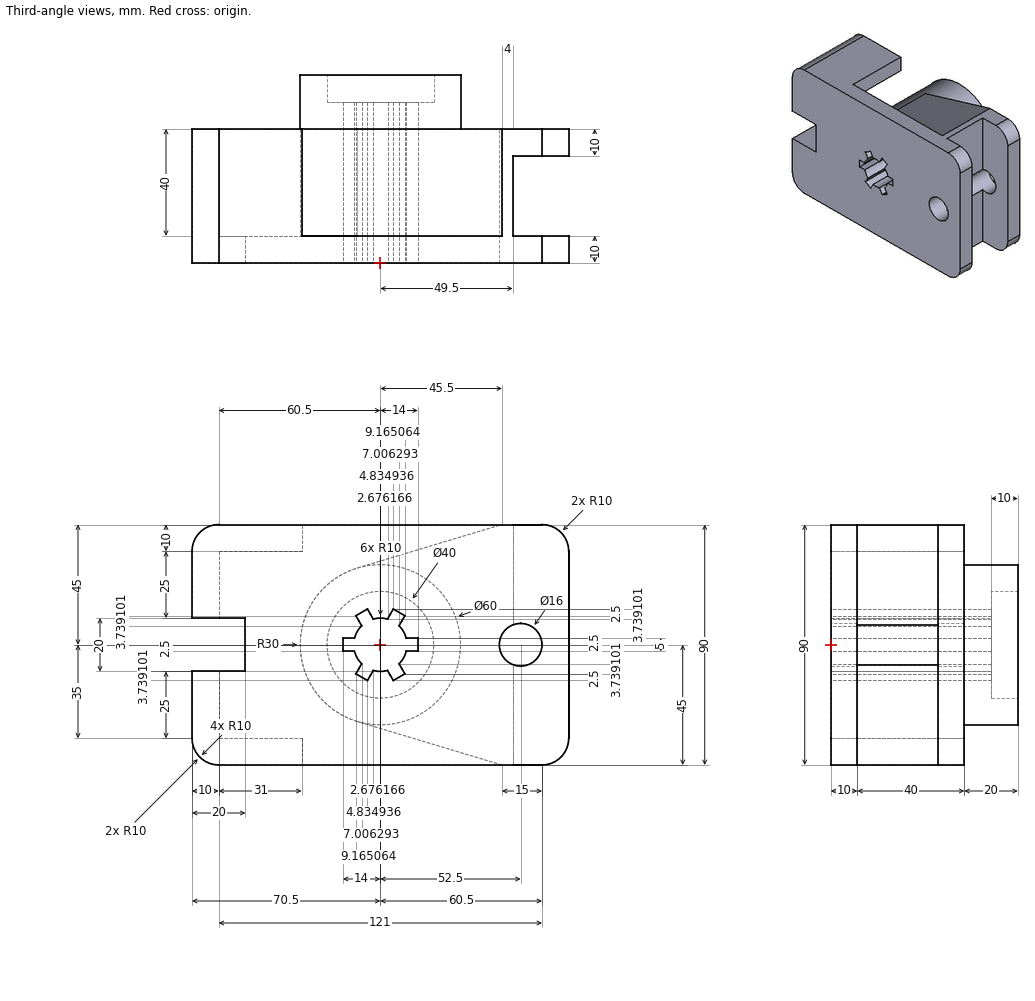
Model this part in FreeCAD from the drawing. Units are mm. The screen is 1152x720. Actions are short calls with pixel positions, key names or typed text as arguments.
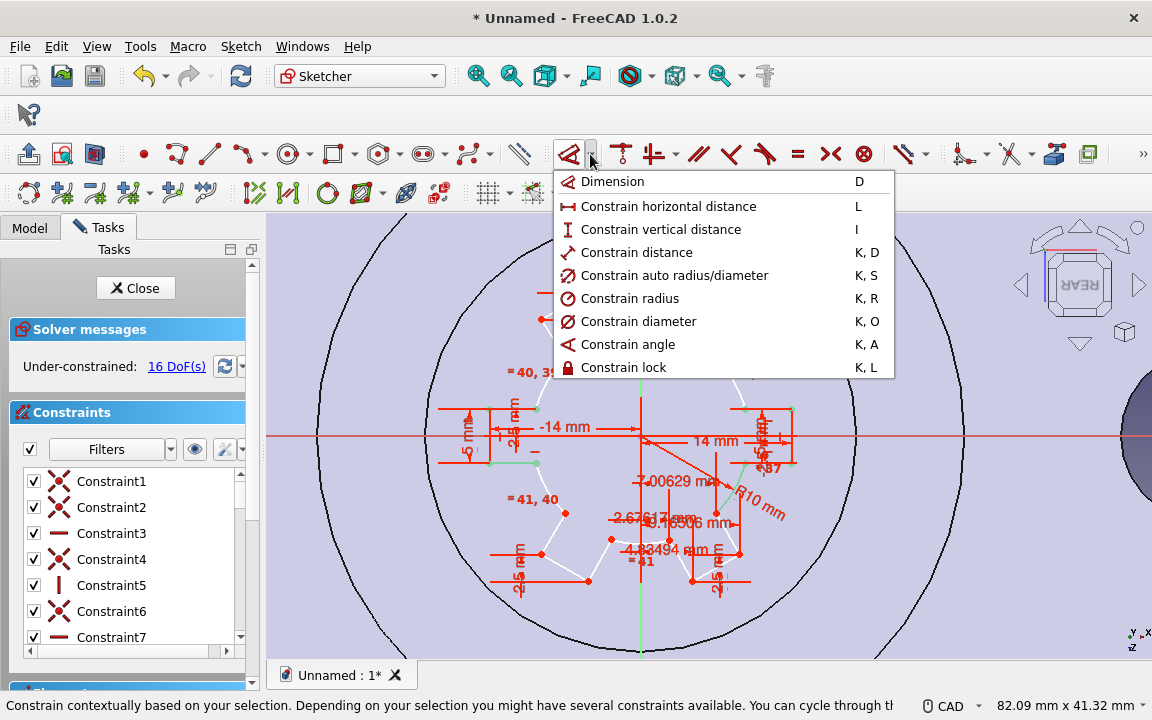
click(724, 206)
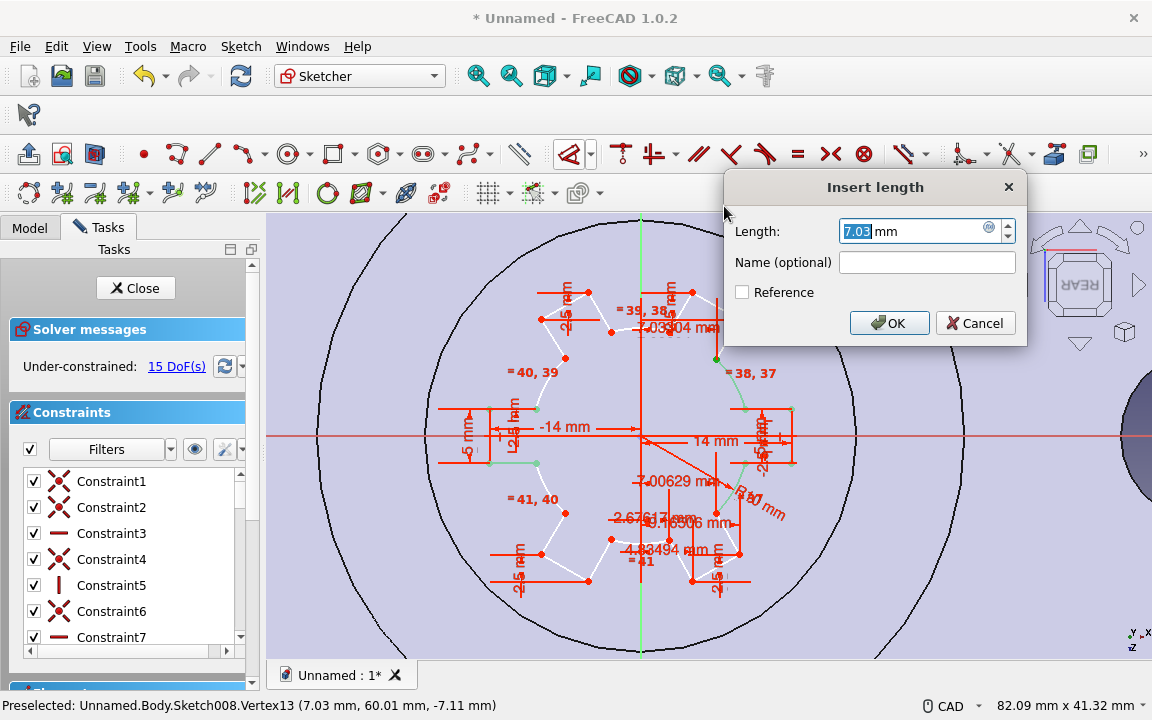
text(7.006293)
key(Return)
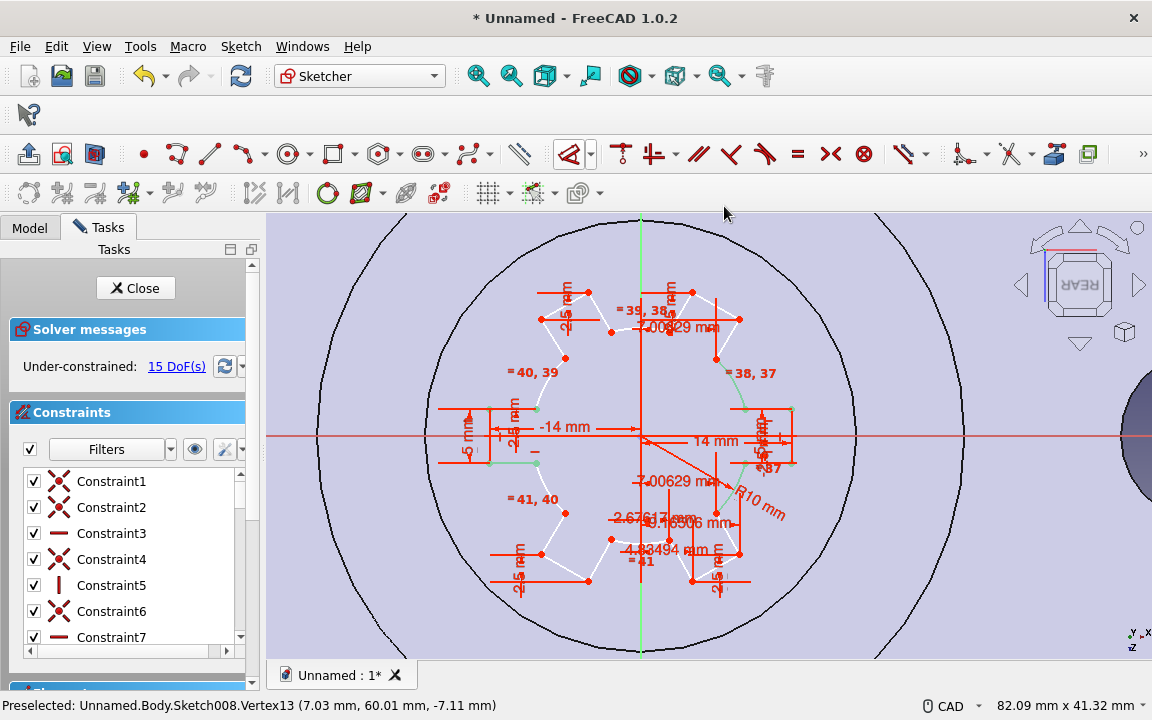
click(739, 320)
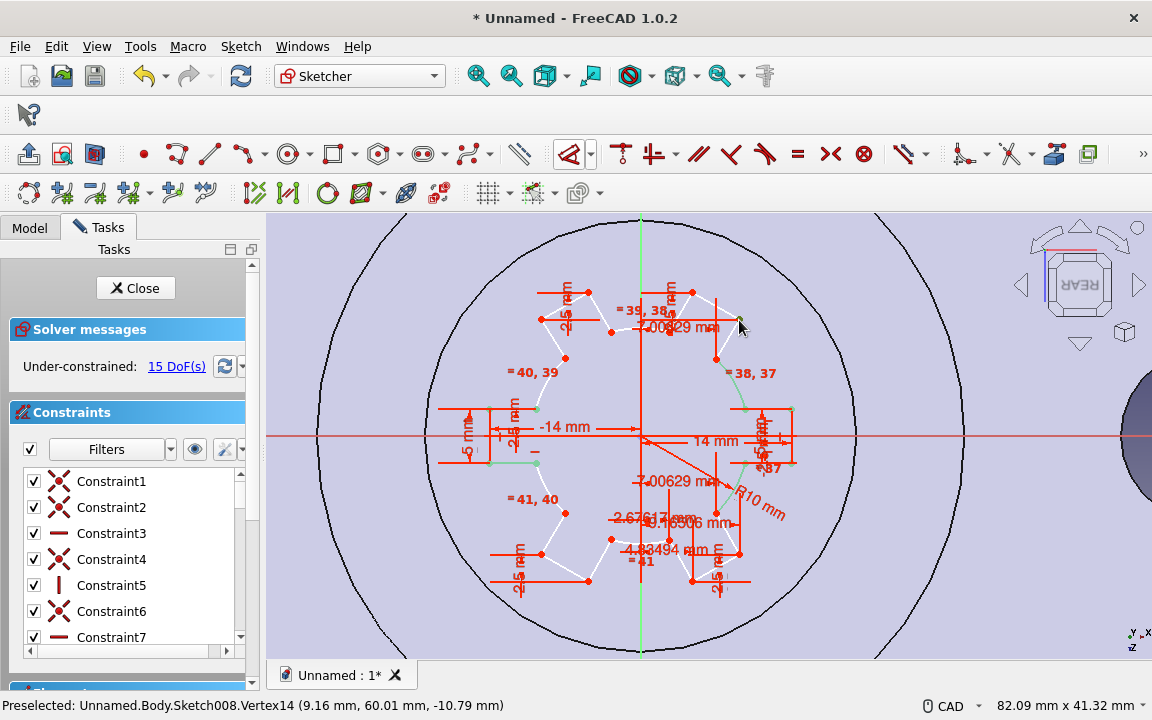
click(590, 154)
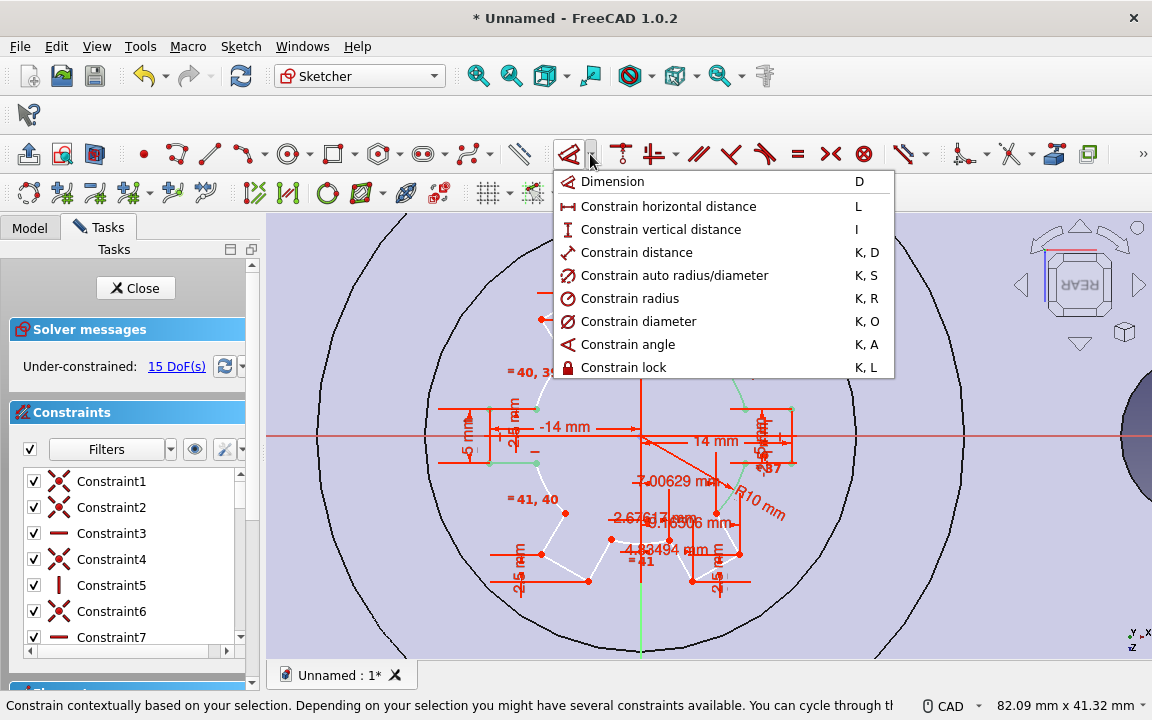
click(724, 206)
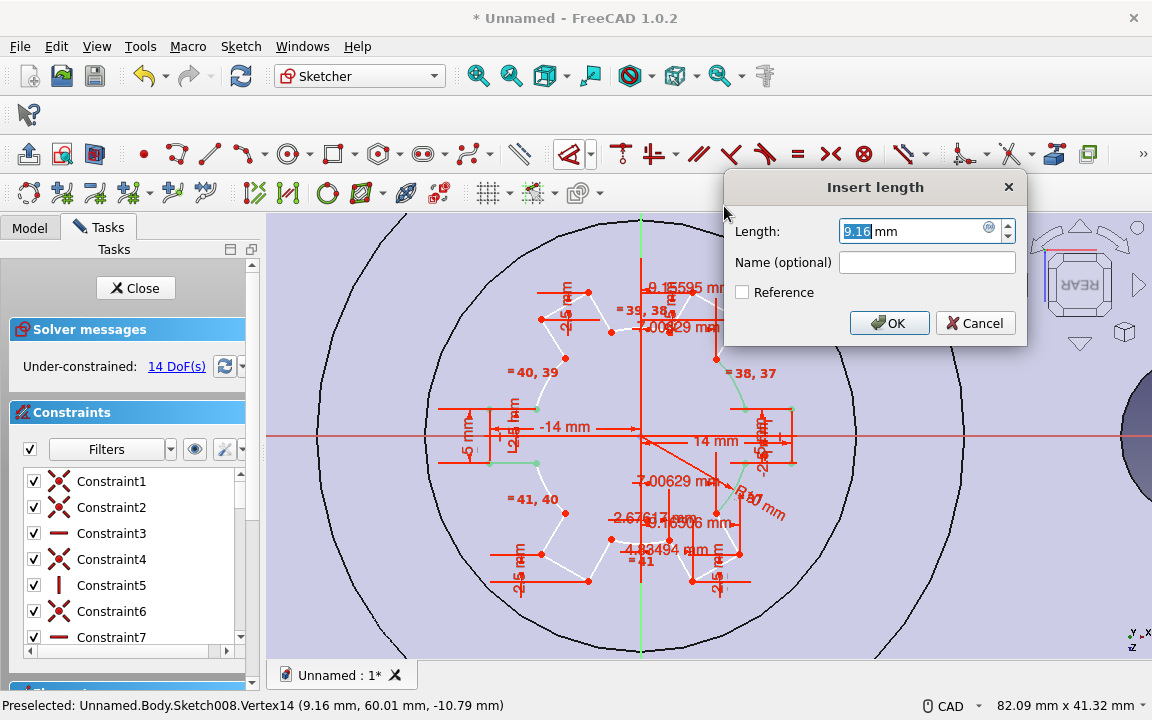
text(9.165064)
key(Return)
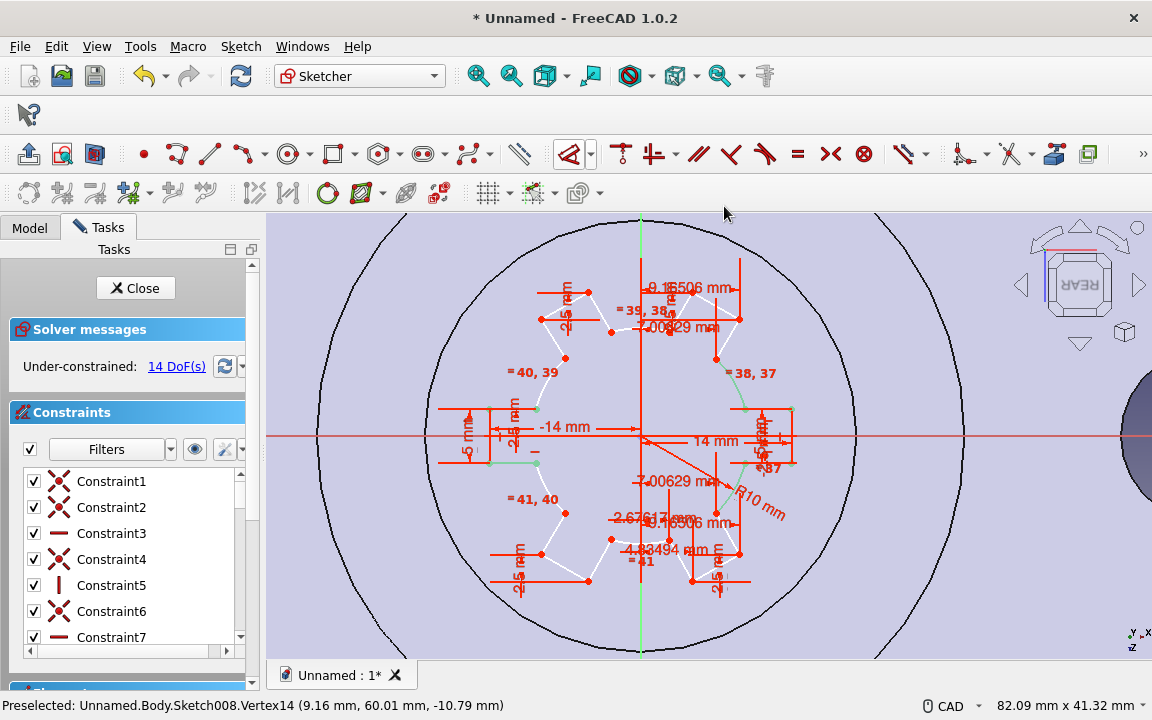
click(692, 293)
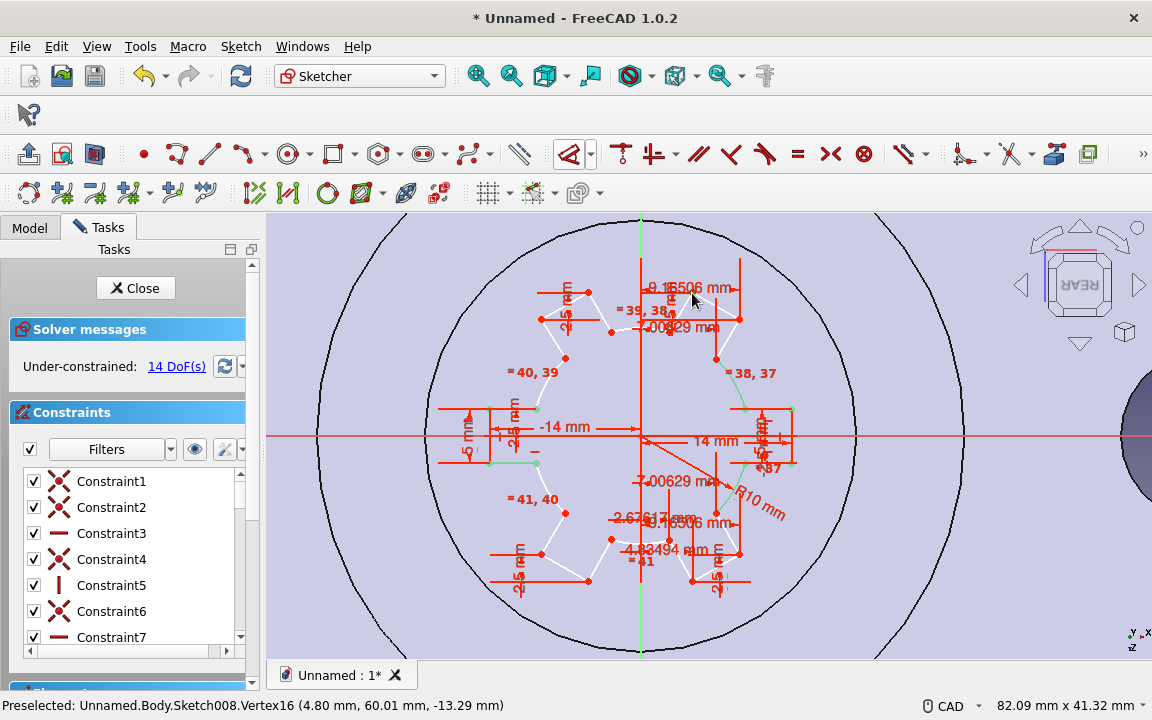
click(590, 154)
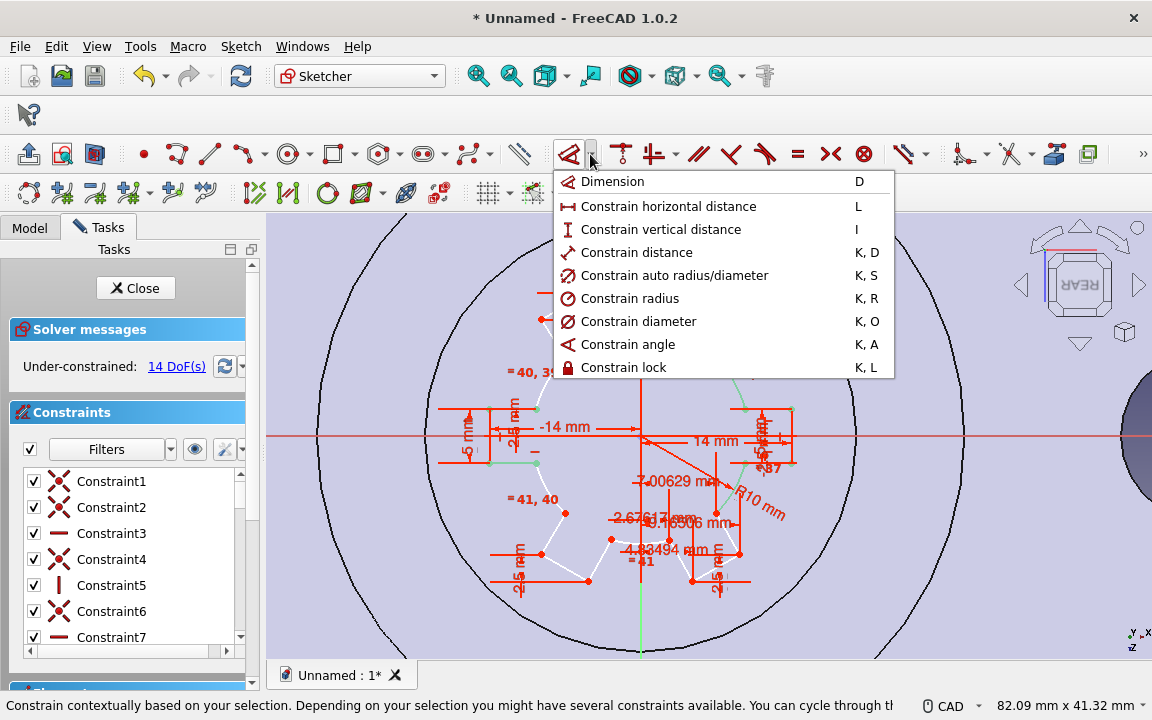
click(724, 206)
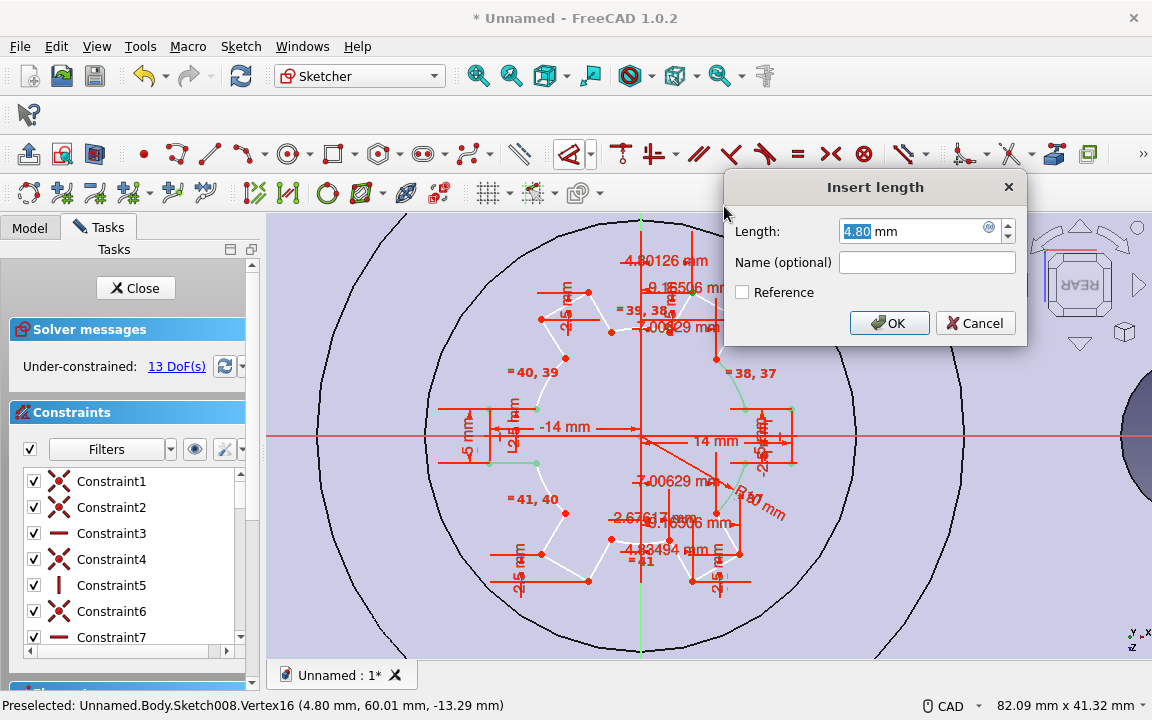
text(4.834936)
key(Return)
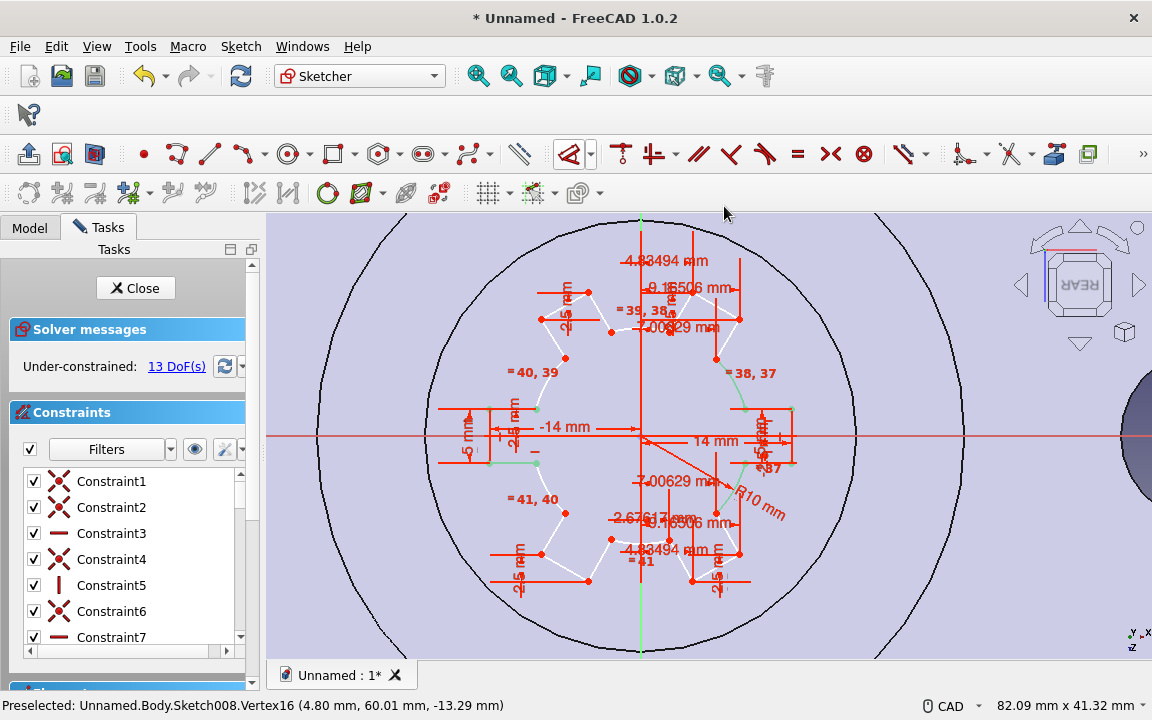
scroll(669, 332, up, 2)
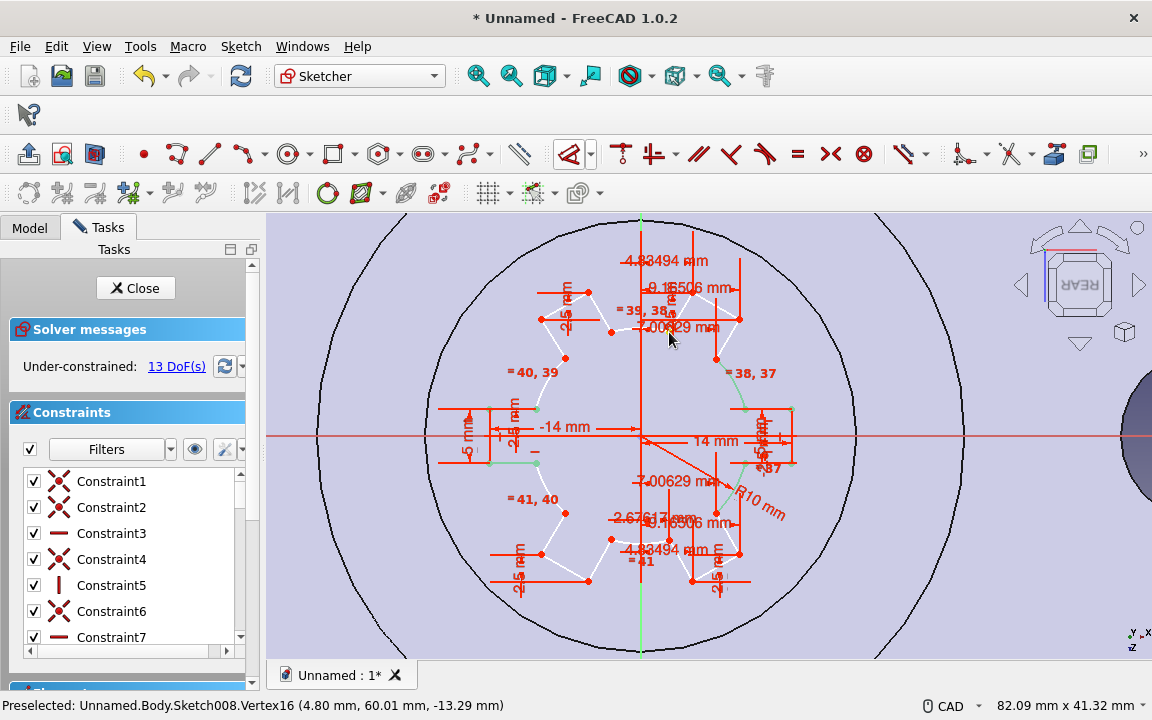
click(669, 332)